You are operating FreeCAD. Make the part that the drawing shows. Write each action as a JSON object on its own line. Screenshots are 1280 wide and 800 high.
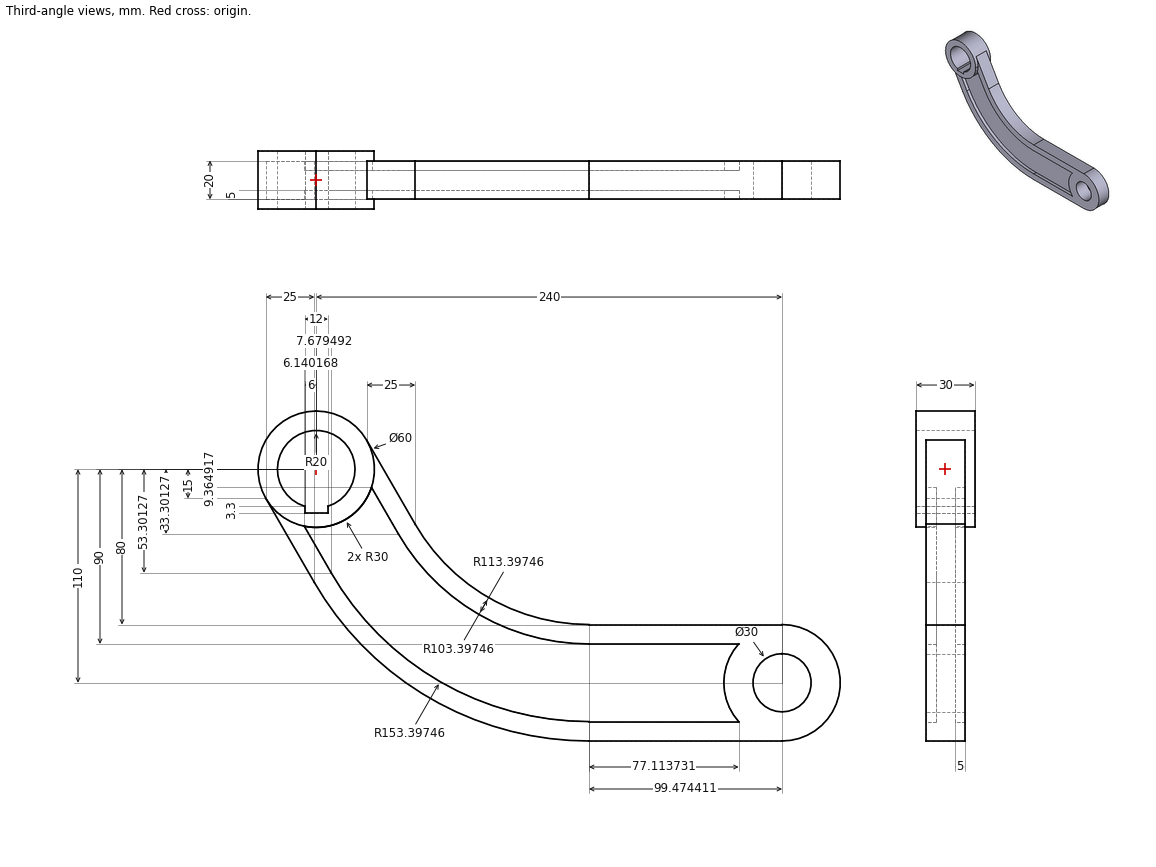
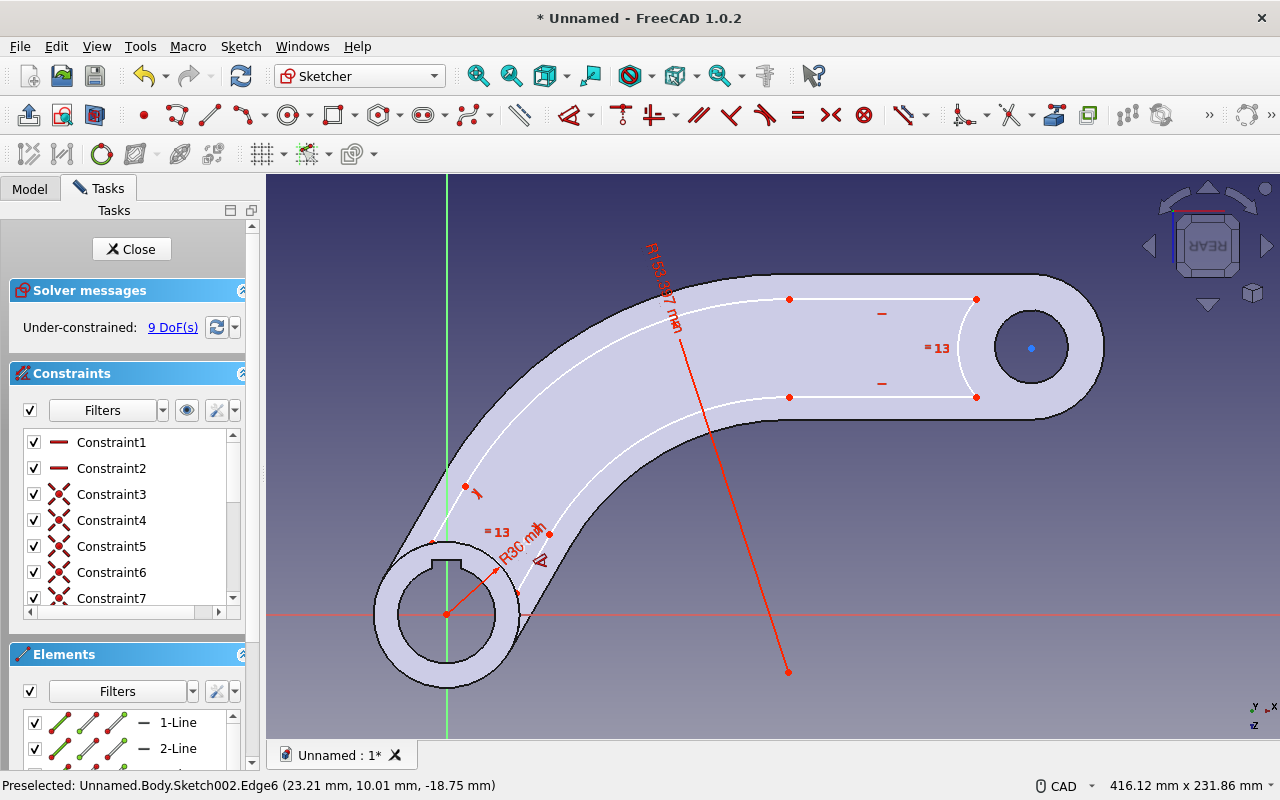
{"action": "left_click", "coordinate": [704, 411]}
{"action": "left_click", "coordinate": [694, 381]}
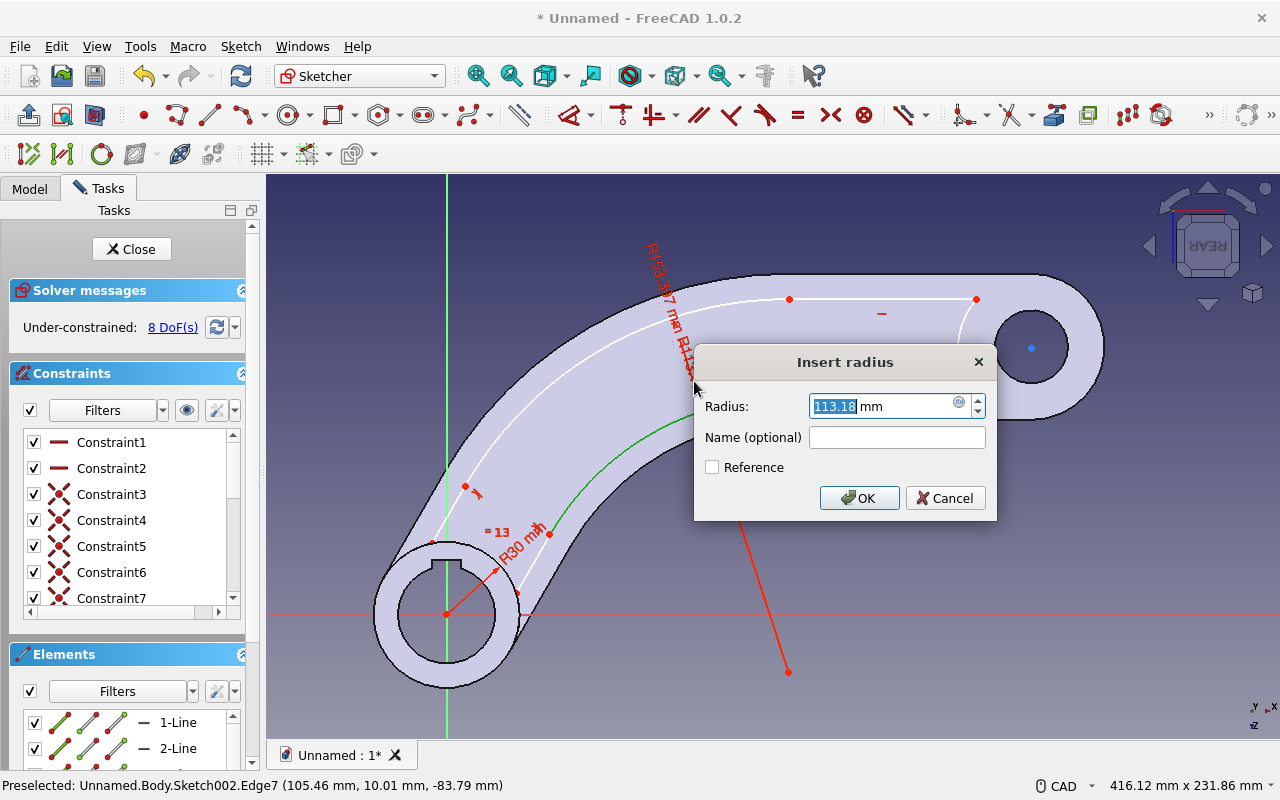
{"action": "type", "text": "113.39746"}
{"action": "key", "text": "Return"}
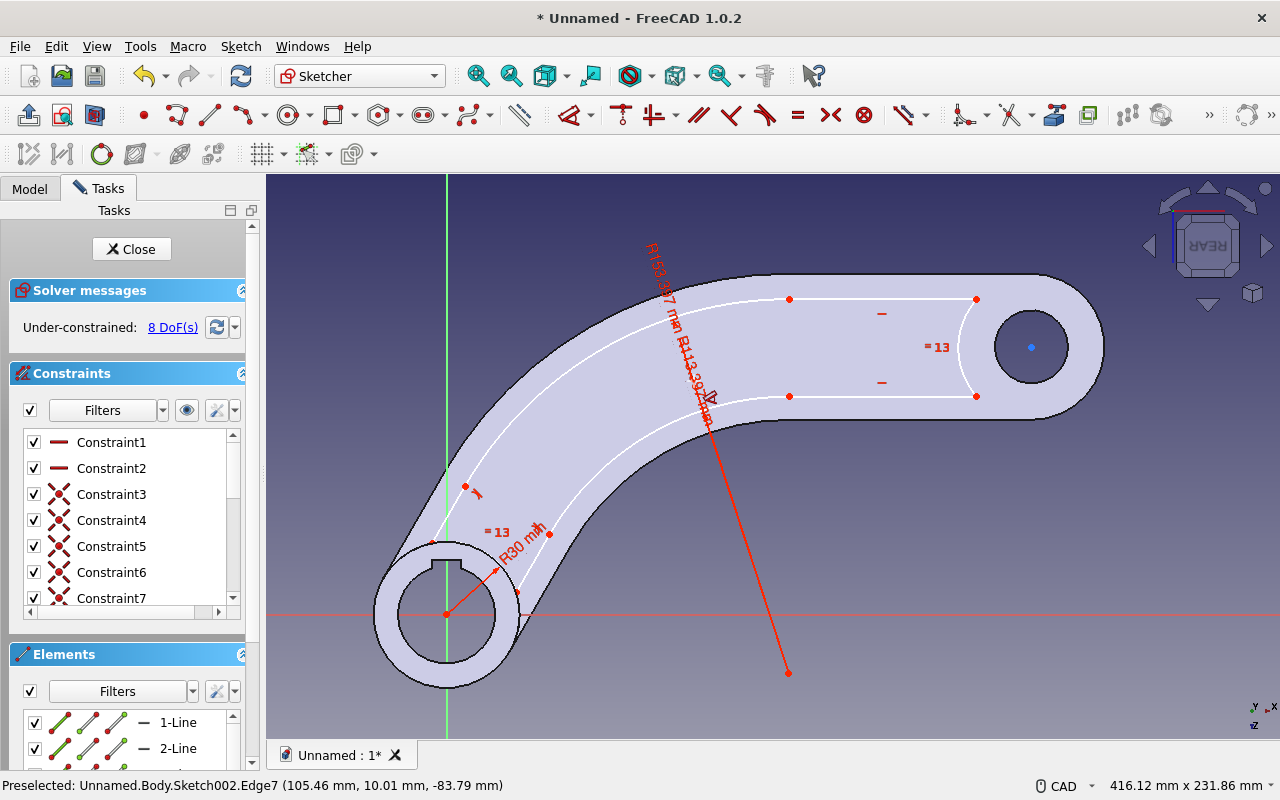
{"action": "left_click", "coordinate": [789, 397]}
{"action": "left_click", "coordinate": [413, 506]}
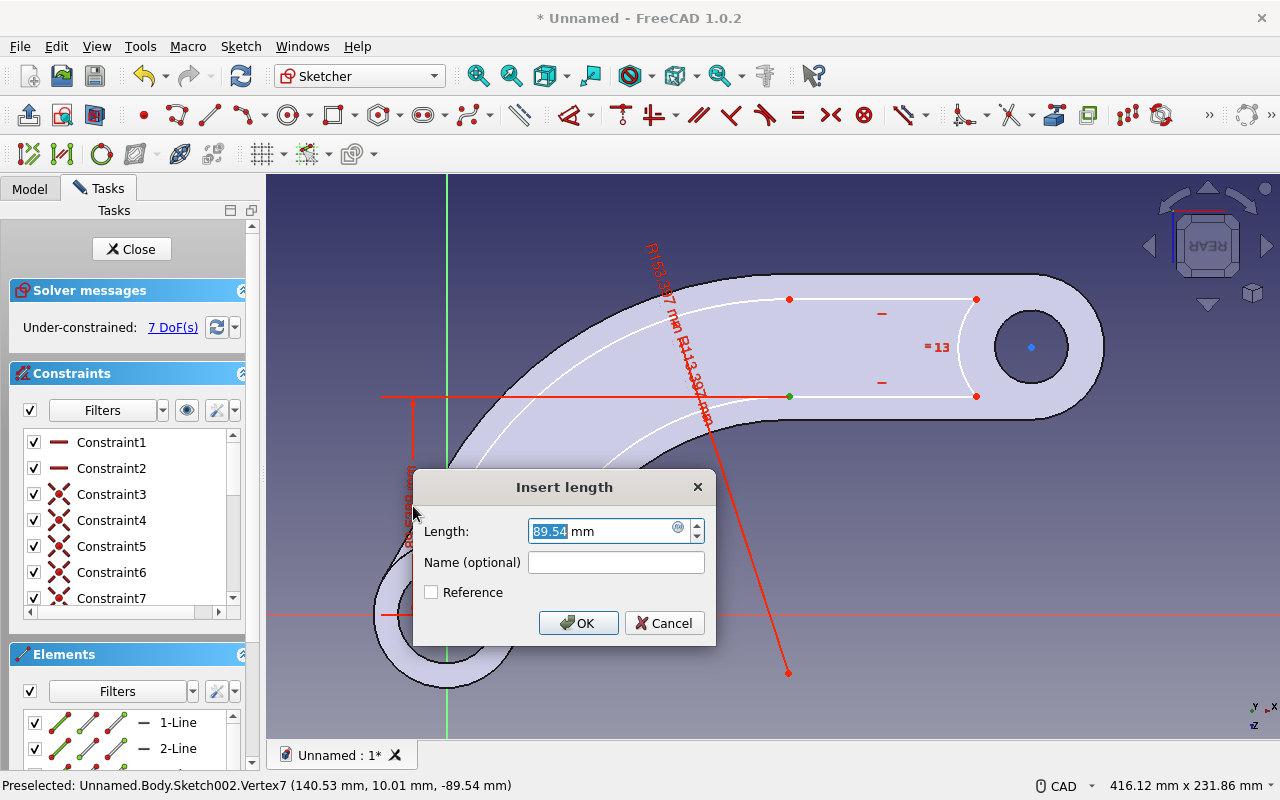
{"action": "type", "text": "90"}
{"action": "key", "text": "Return"}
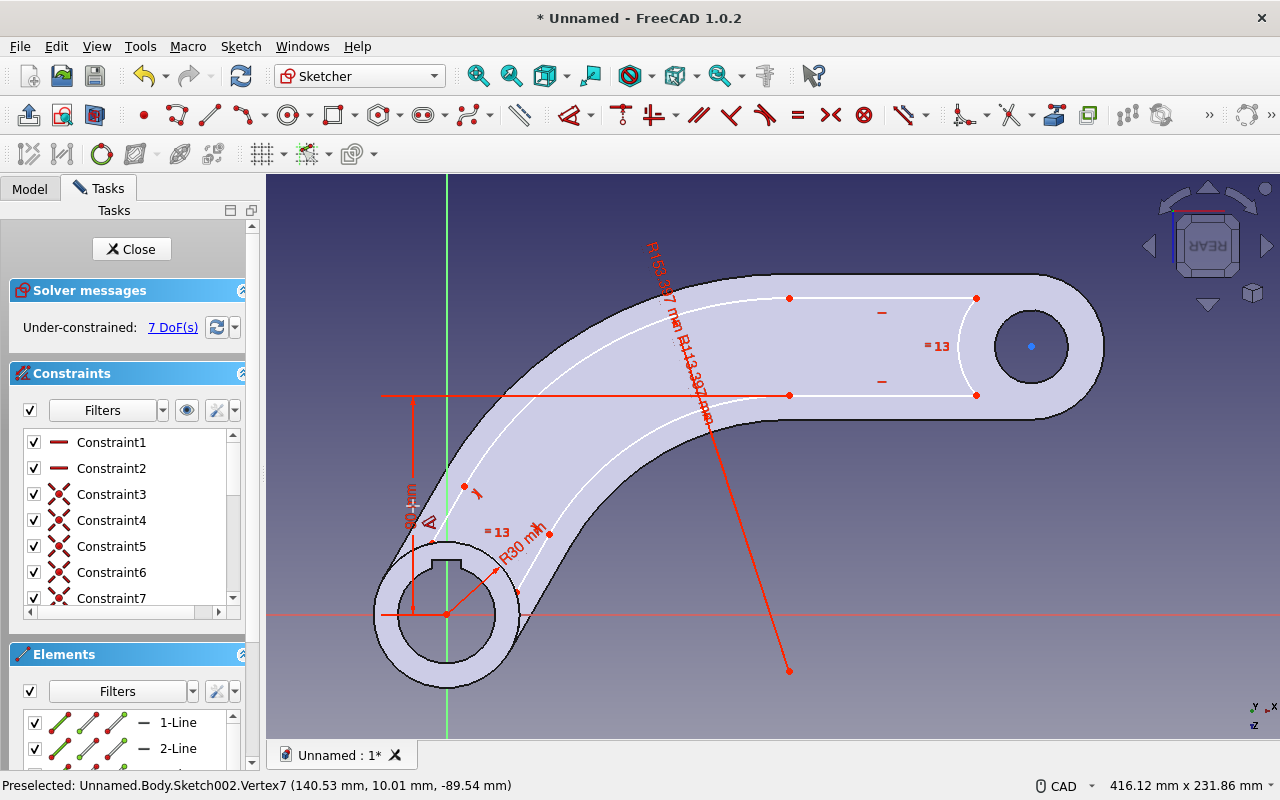
{"action": "left_click", "coordinate": [1031, 347]}
{"action": "left_click", "coordinate": [739, 649]}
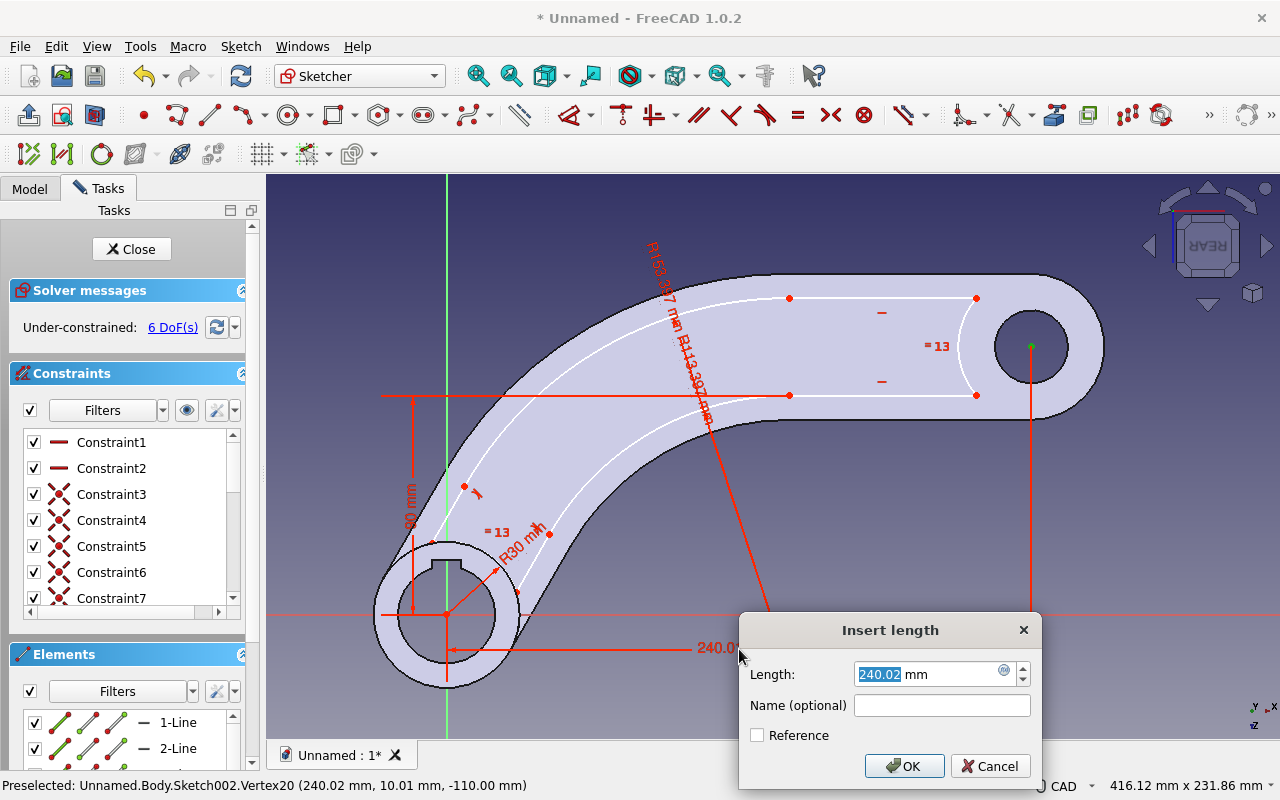
{"action": "type", "text": "240"}
{"action": "key", "text": "Return"}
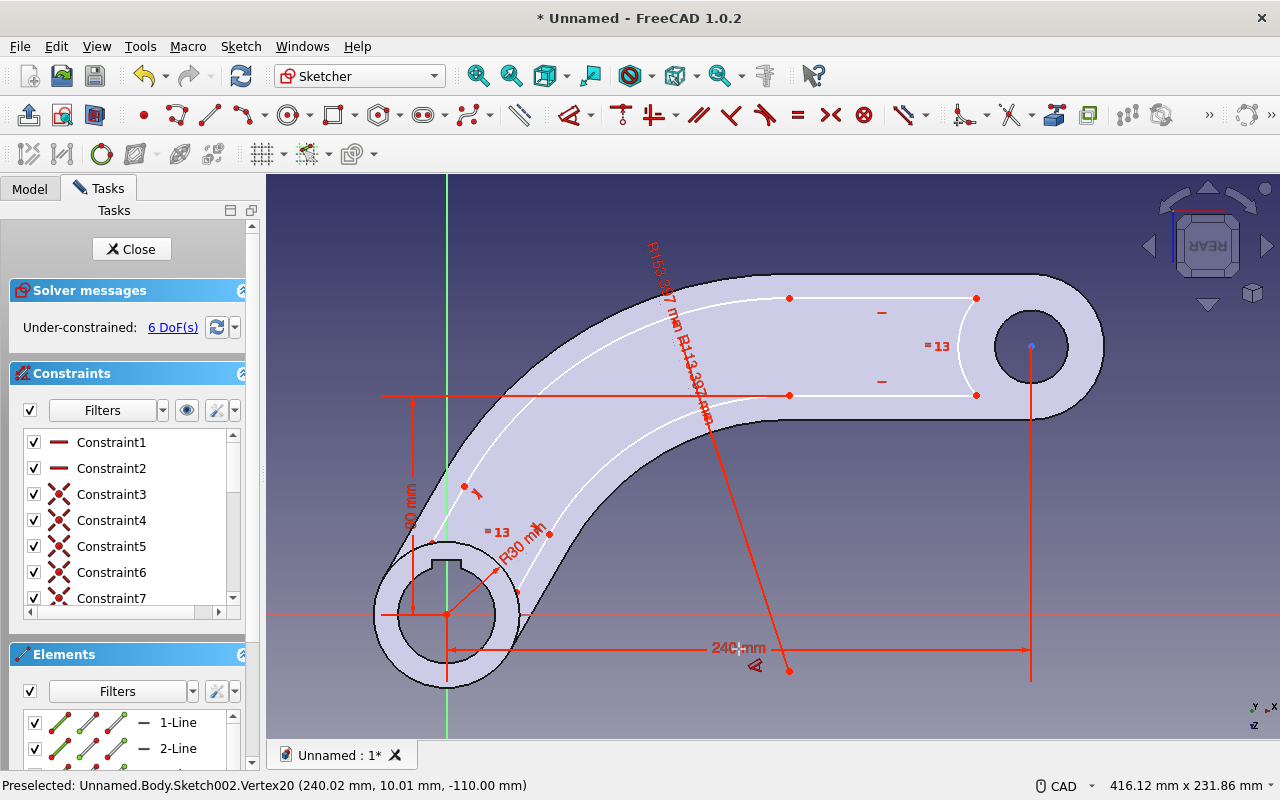
{"action": "left_click", "coordinate": [1031, 347]}
{"action": "left_click", "coordinate": [1065, 481]}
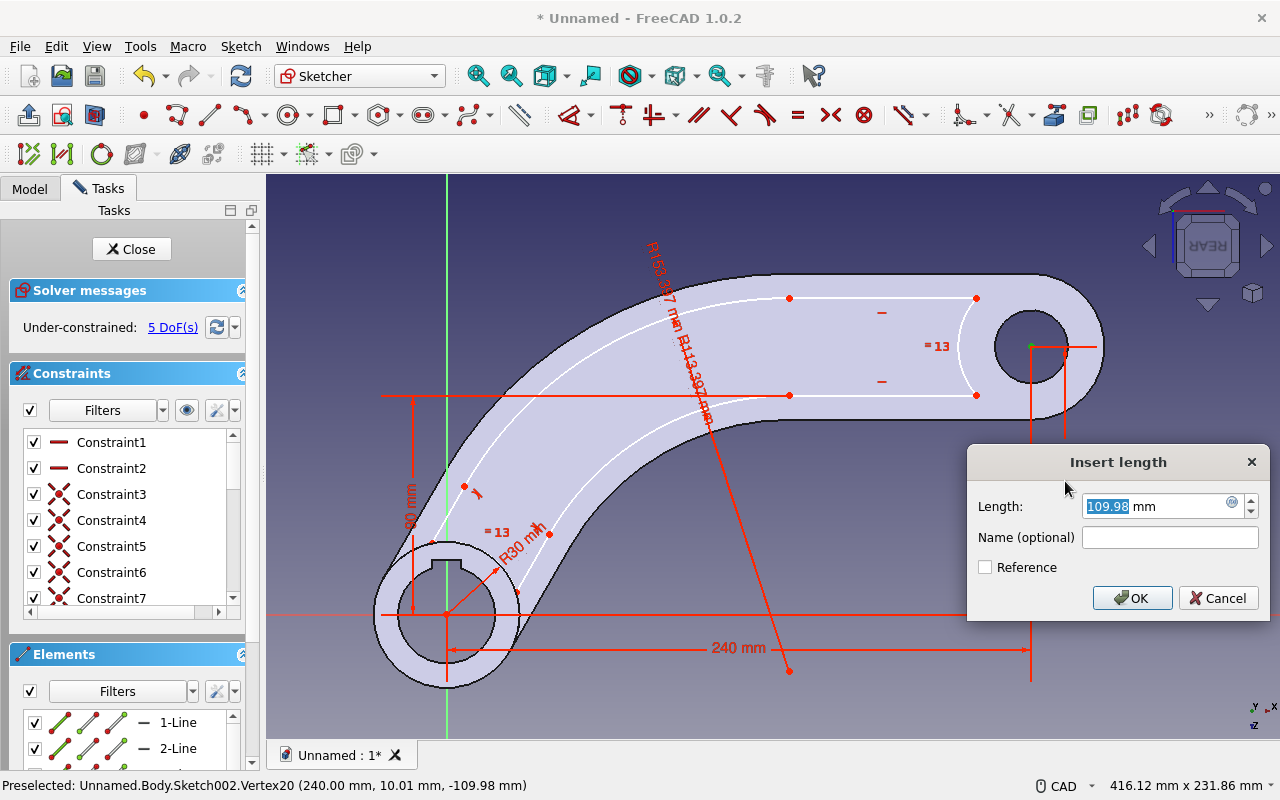
{"action": "type", "text": "110"}
{"action": "key", "text": "Return"}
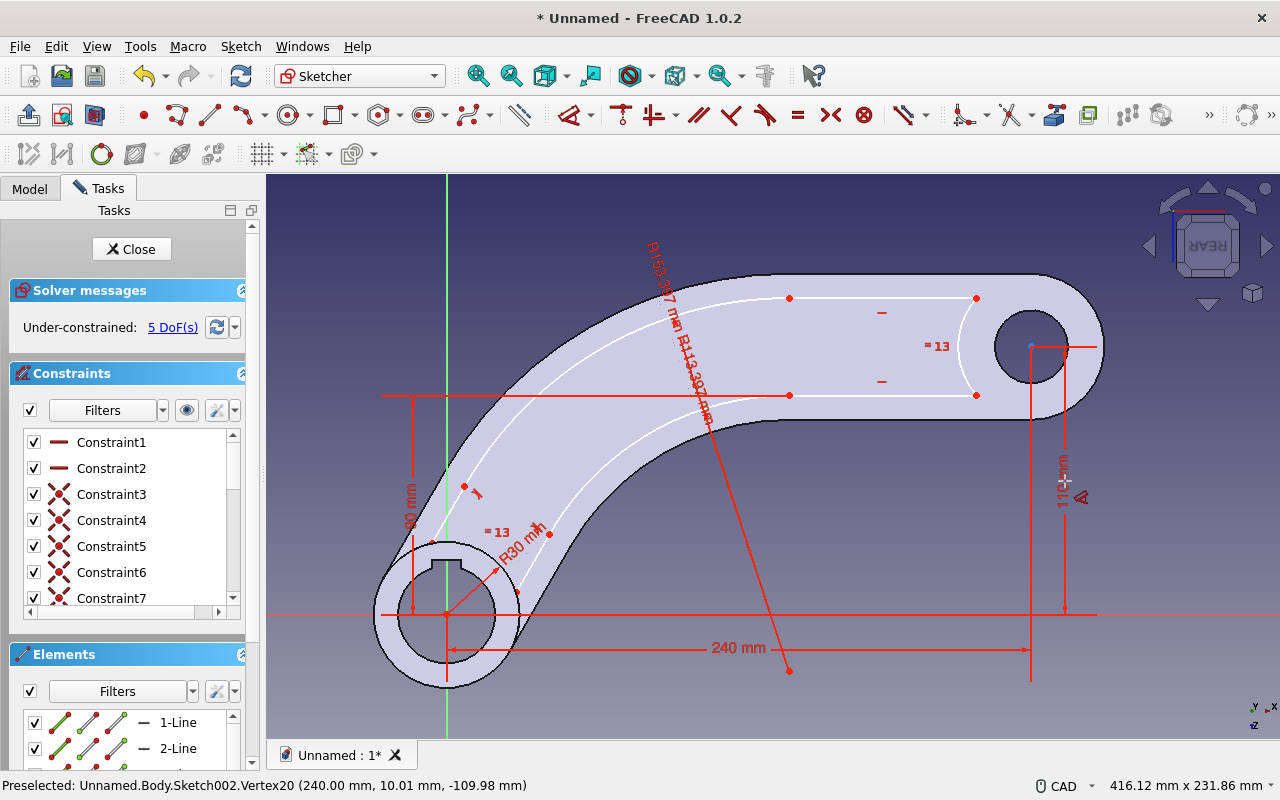
{"action": "left_click", "coordinate": [921, 298]}
{"action": "left_click", "coordinate": [883, 264]}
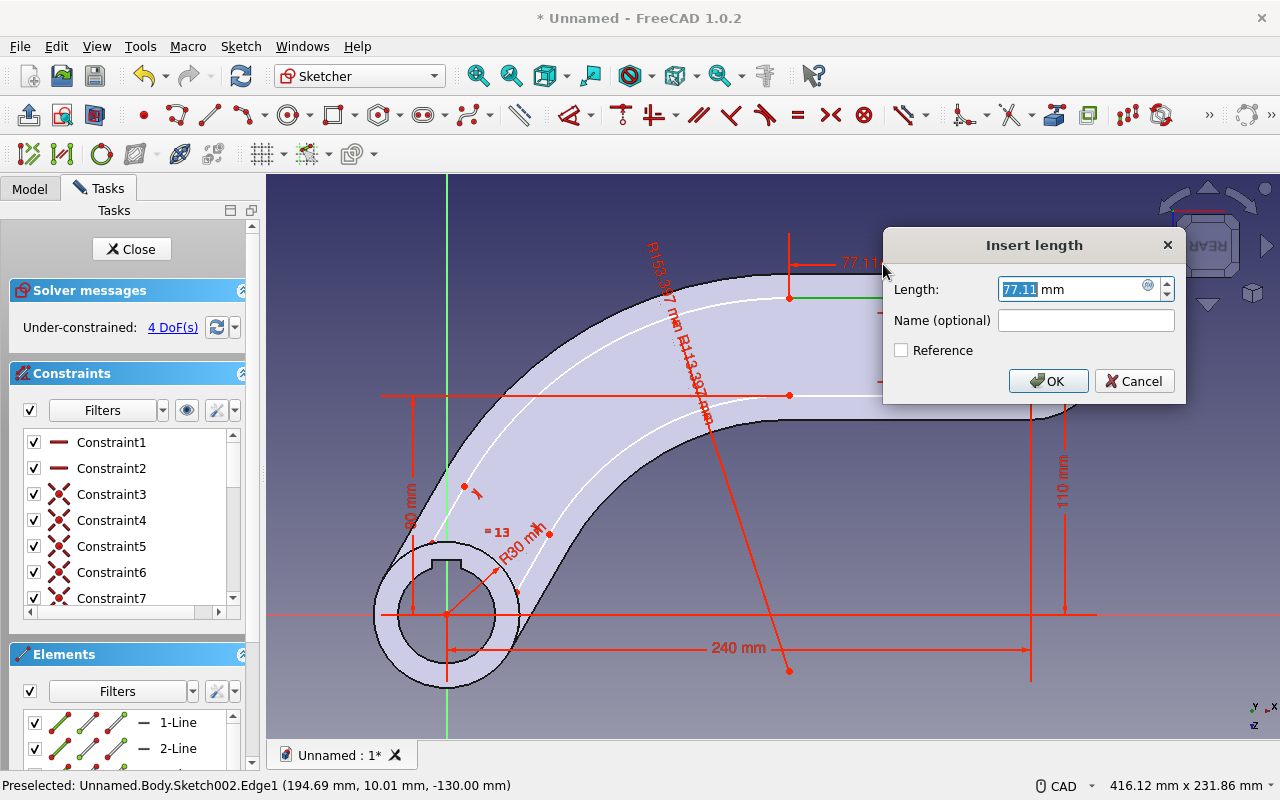
{"action": "type", "text": "77.113731"}
{"action": "key", "text": "Return"}